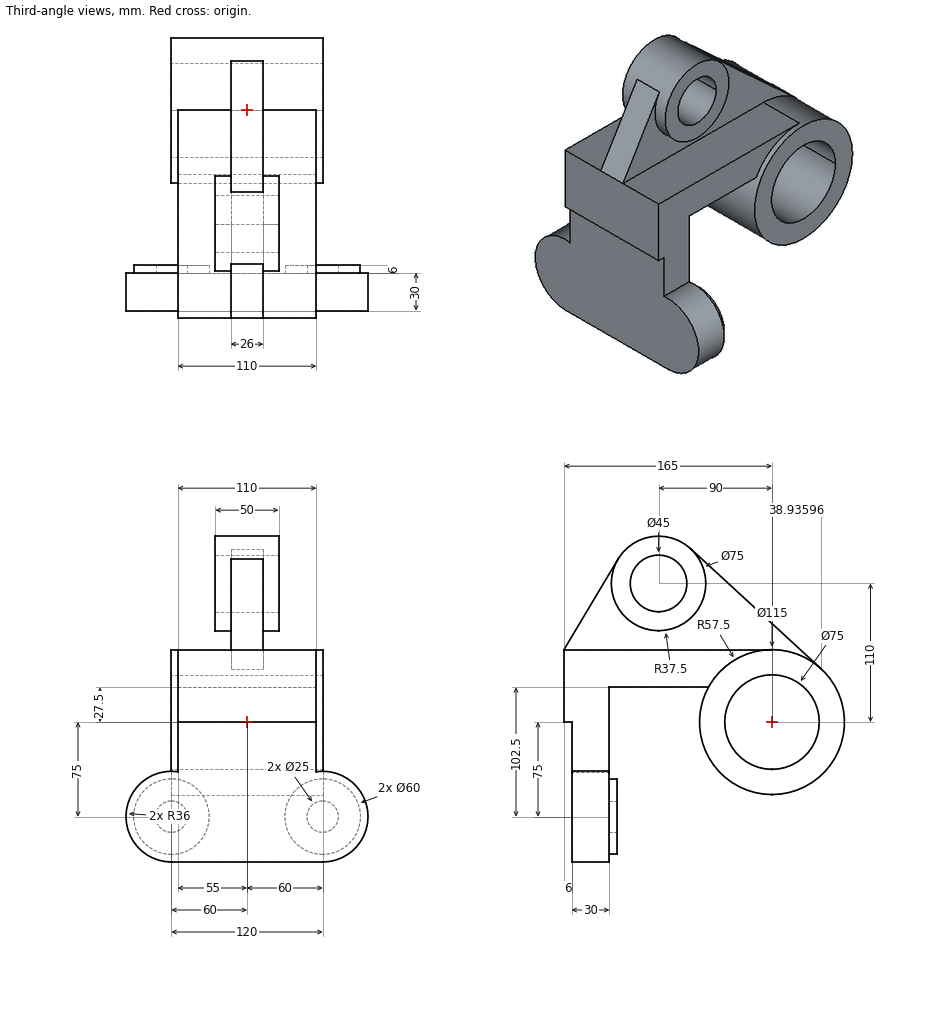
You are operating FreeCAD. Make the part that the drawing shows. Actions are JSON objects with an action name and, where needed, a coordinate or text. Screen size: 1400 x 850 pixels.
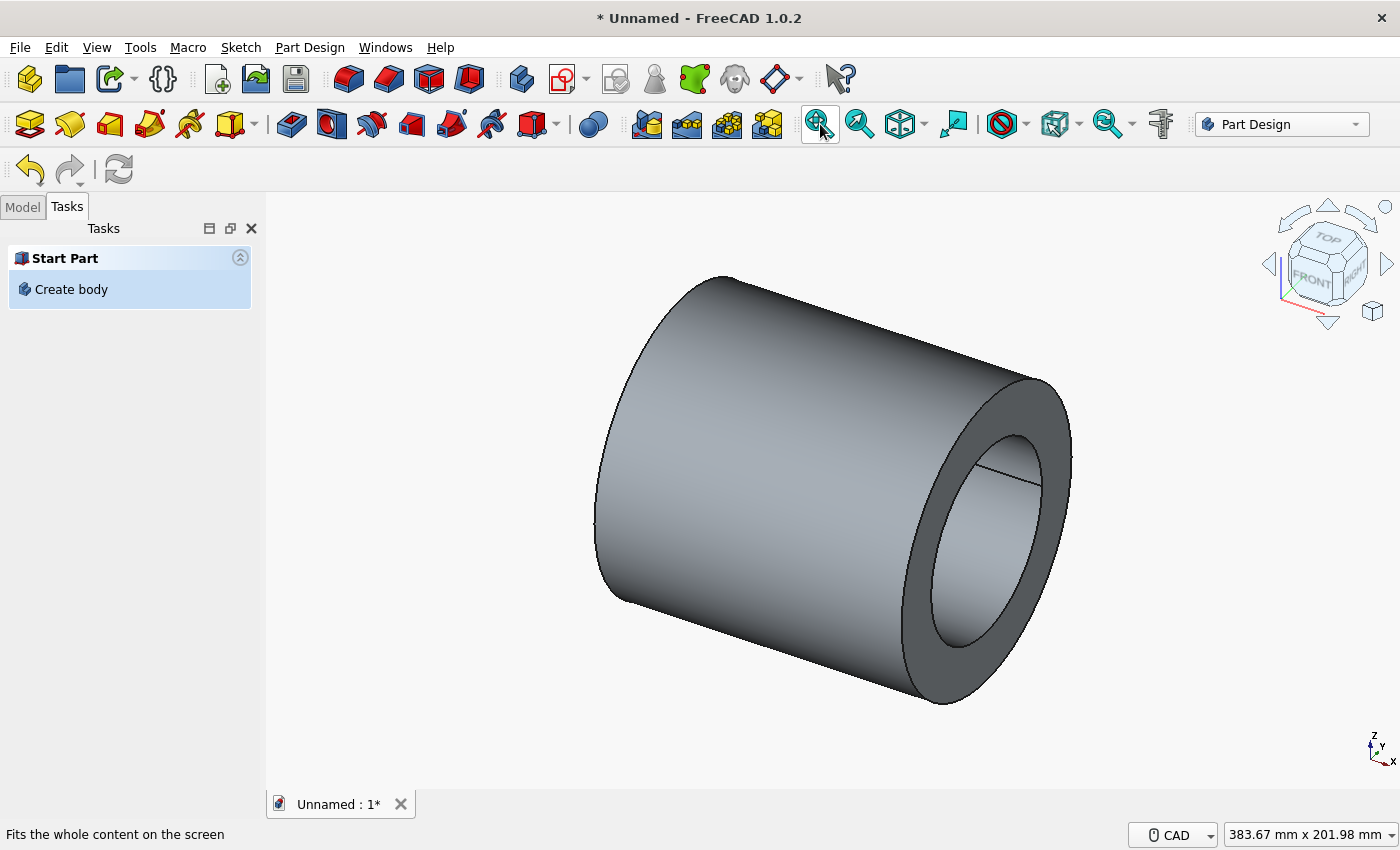
{"action": "left_click", "coordinate": [562, 80]}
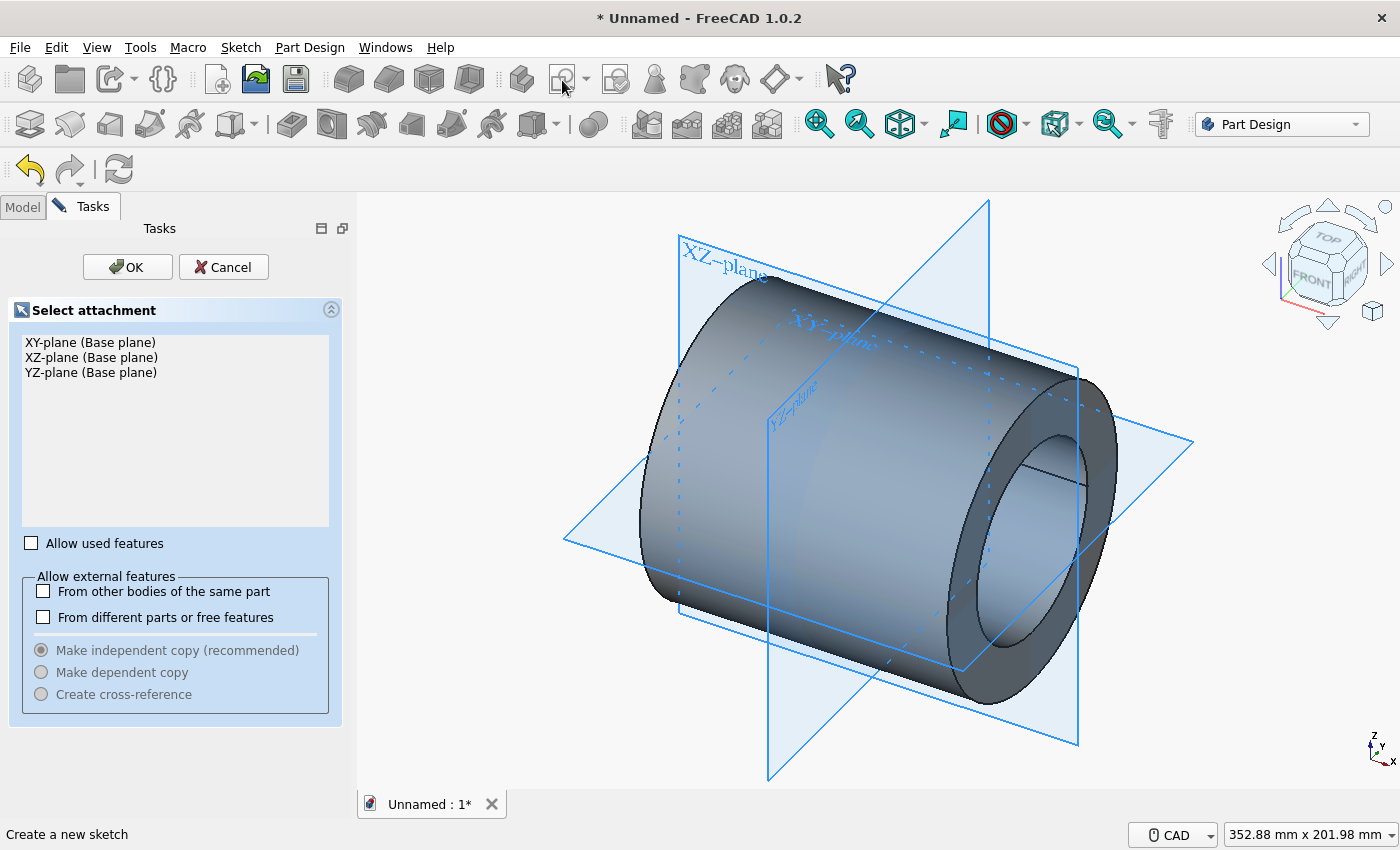
{"action": "left_click", "coordinate": [82, 372]}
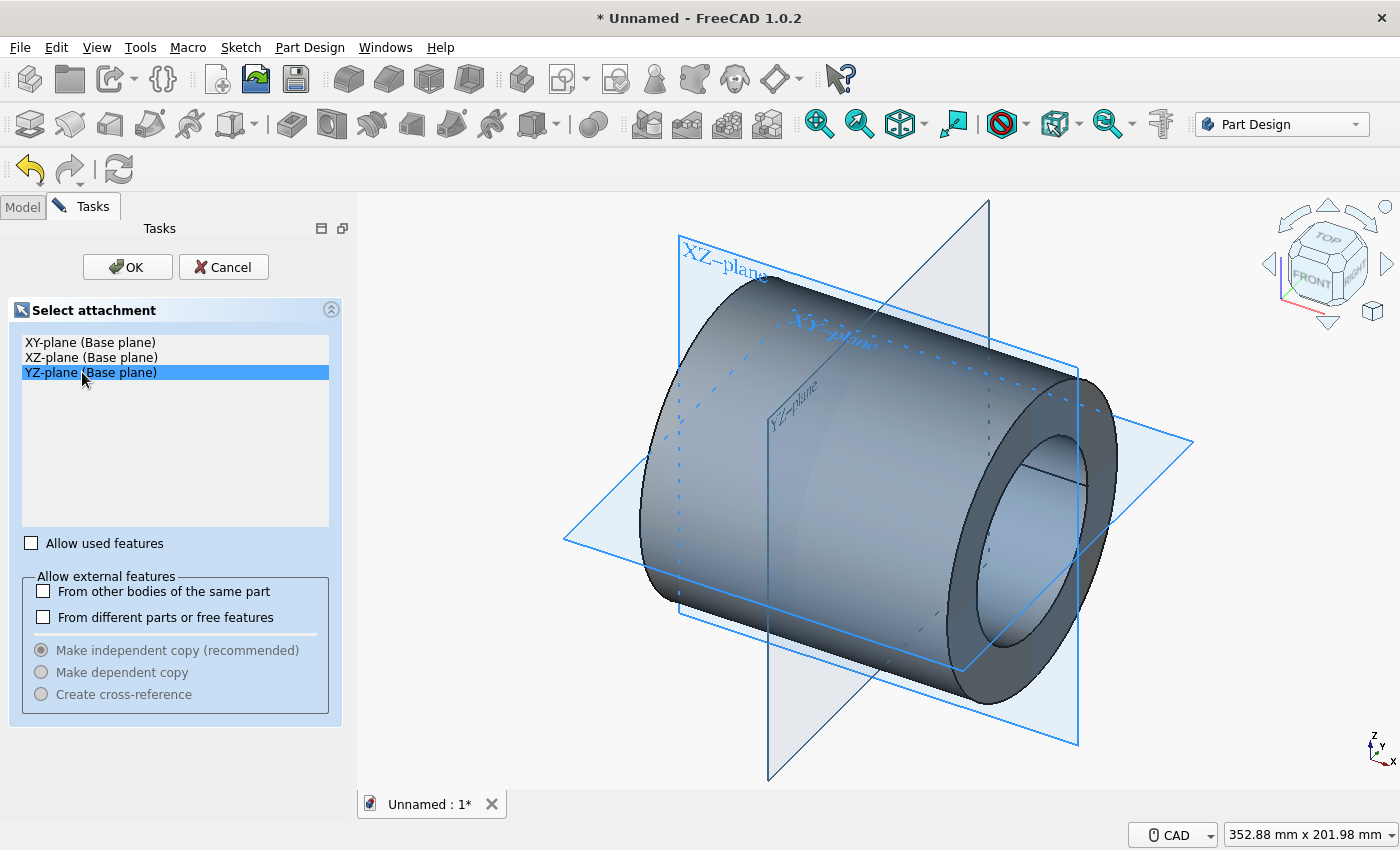
{"action": "left_click", "coordinate": [128, 267]}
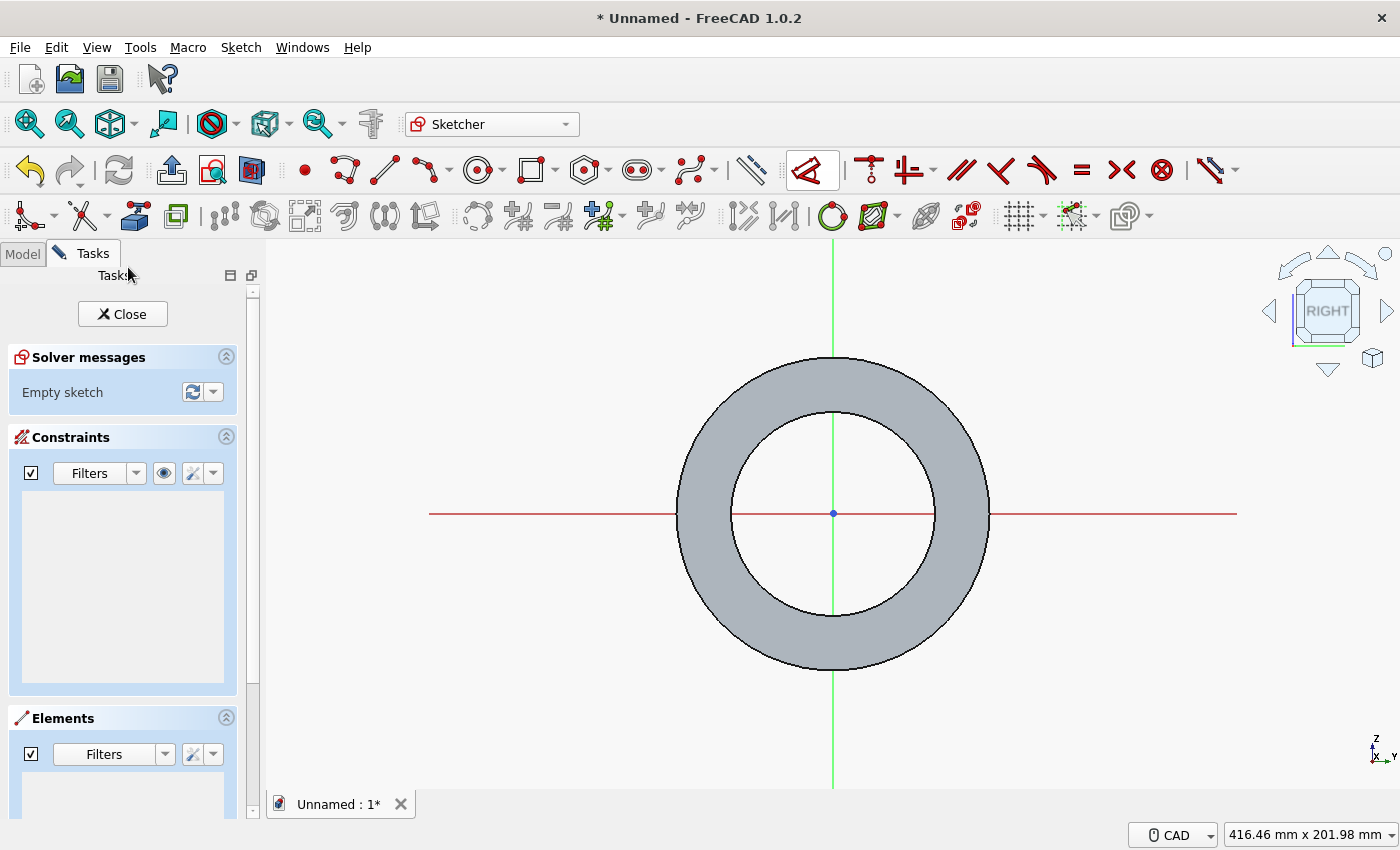
{"action": "left_click", "coordinate": [252, 170]}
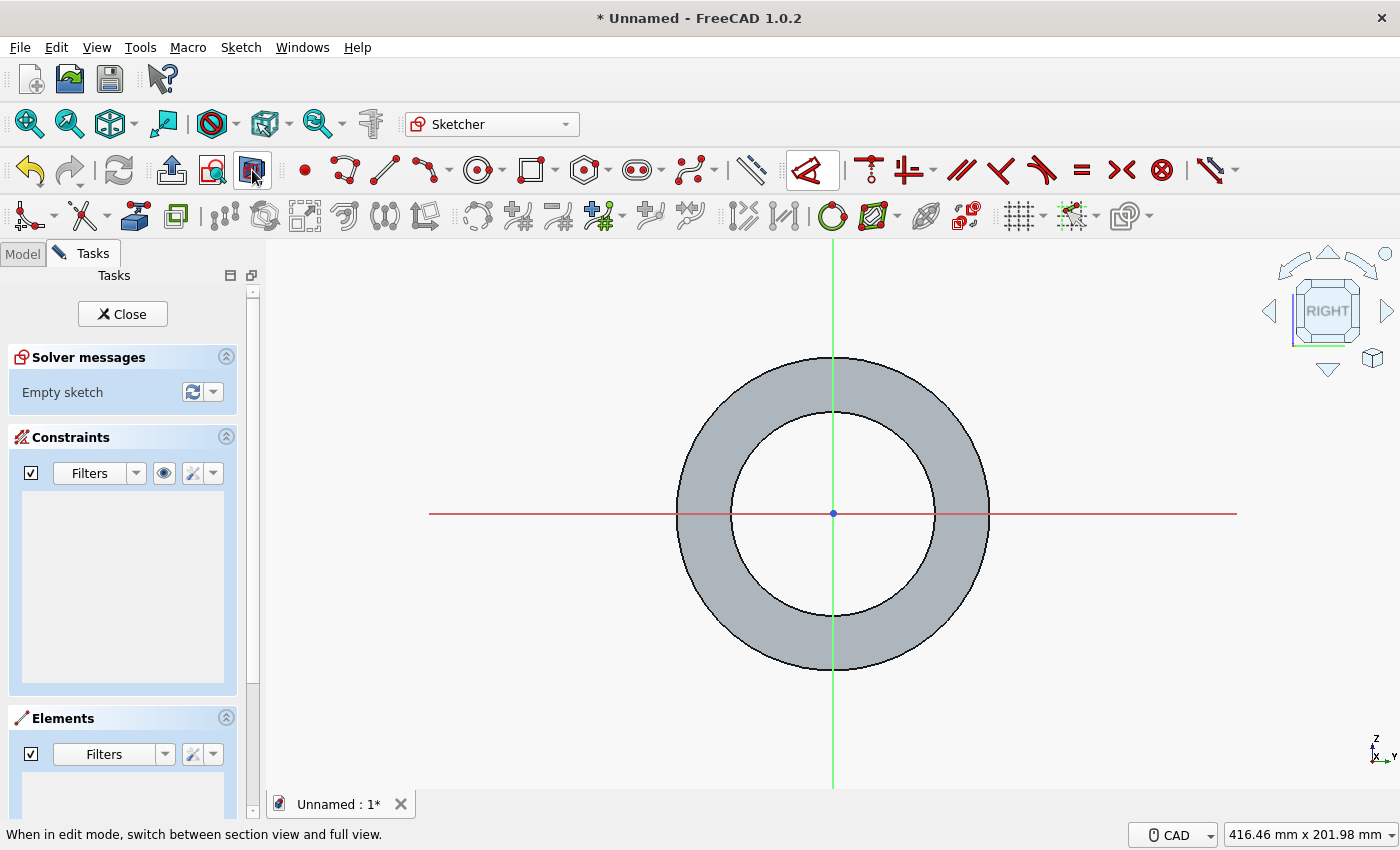
{"action": "key", "text": "g m"}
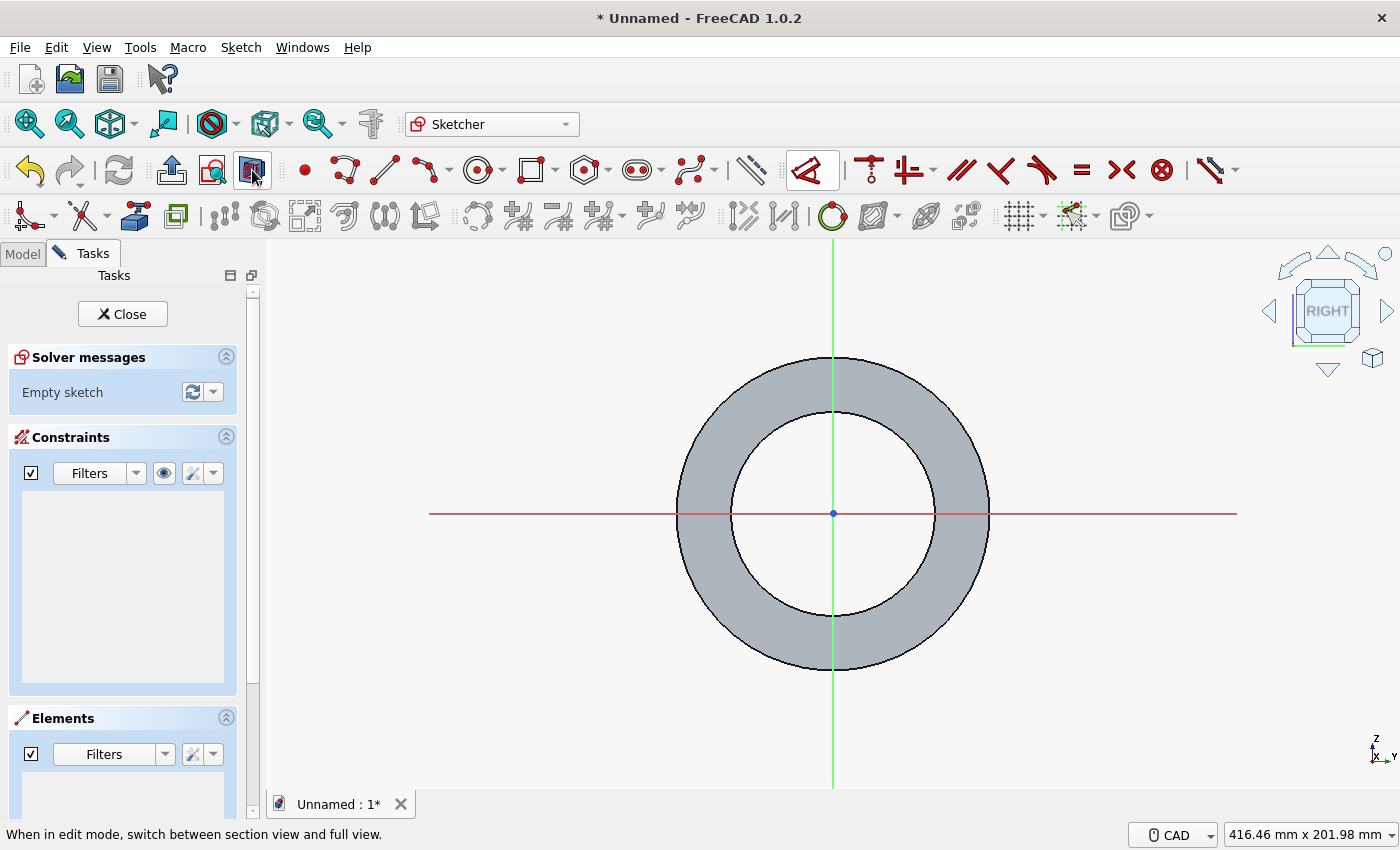
{"action": "left_click", "coordinate": [833, 357]}
{"action": "left_click", "coordinate": [384, 357]}
{"action": "left_click", "coordinate": [384, 514]}
{"action": "left_click", "coordinate": [400, 523]}
{"action": "left_click", "coordinate": [400, 718]}
{"action": "left_click", "coordinate": [482, 718]}
{"action": "left_click", "coordinate": [482, 439]}
{"action": "left_click", "coordinate": [695, 439]}
{"action": "right_click", "coordinate": [695, 439]}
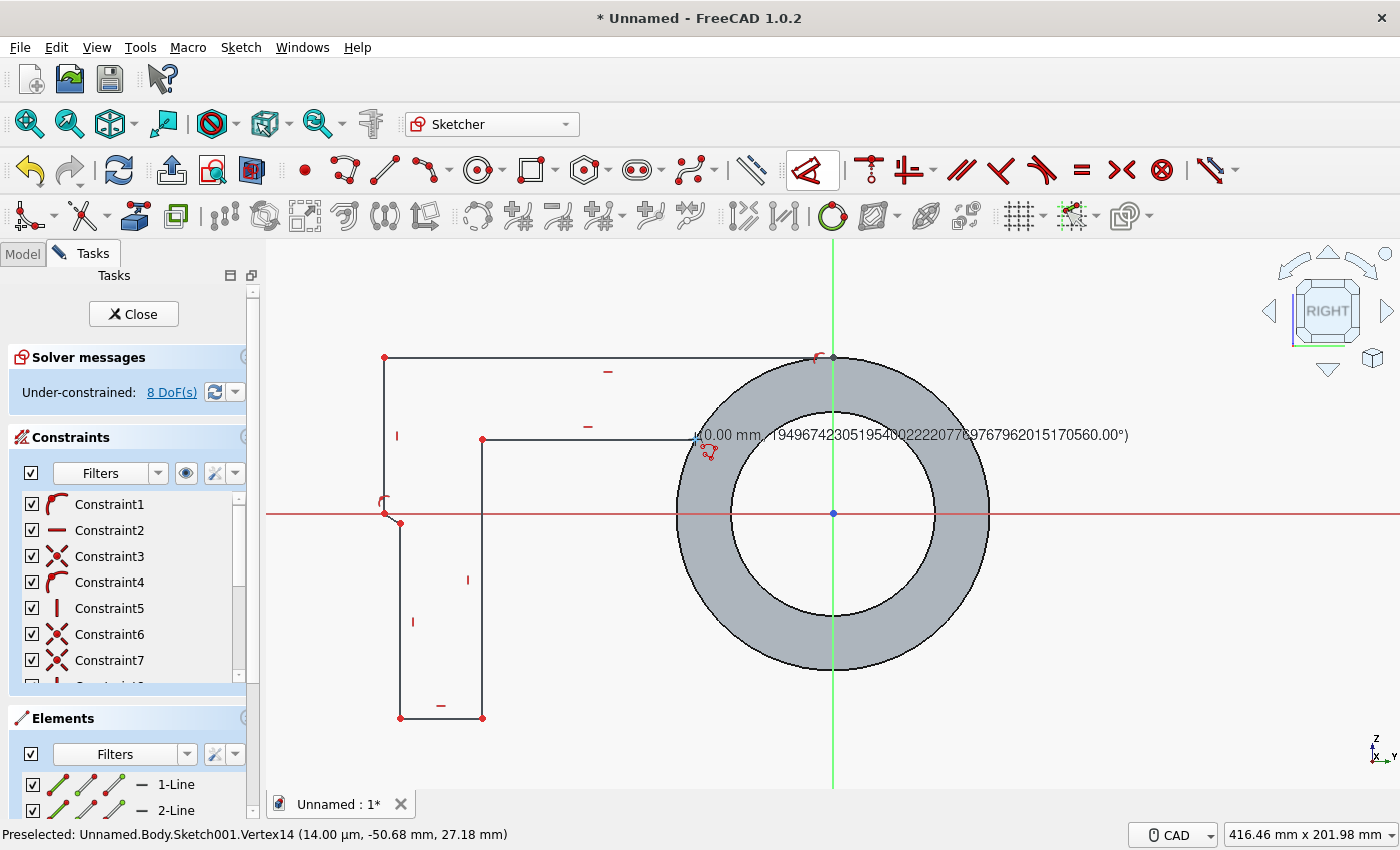
{"action": "left_click", "coordinate": [426, 170]}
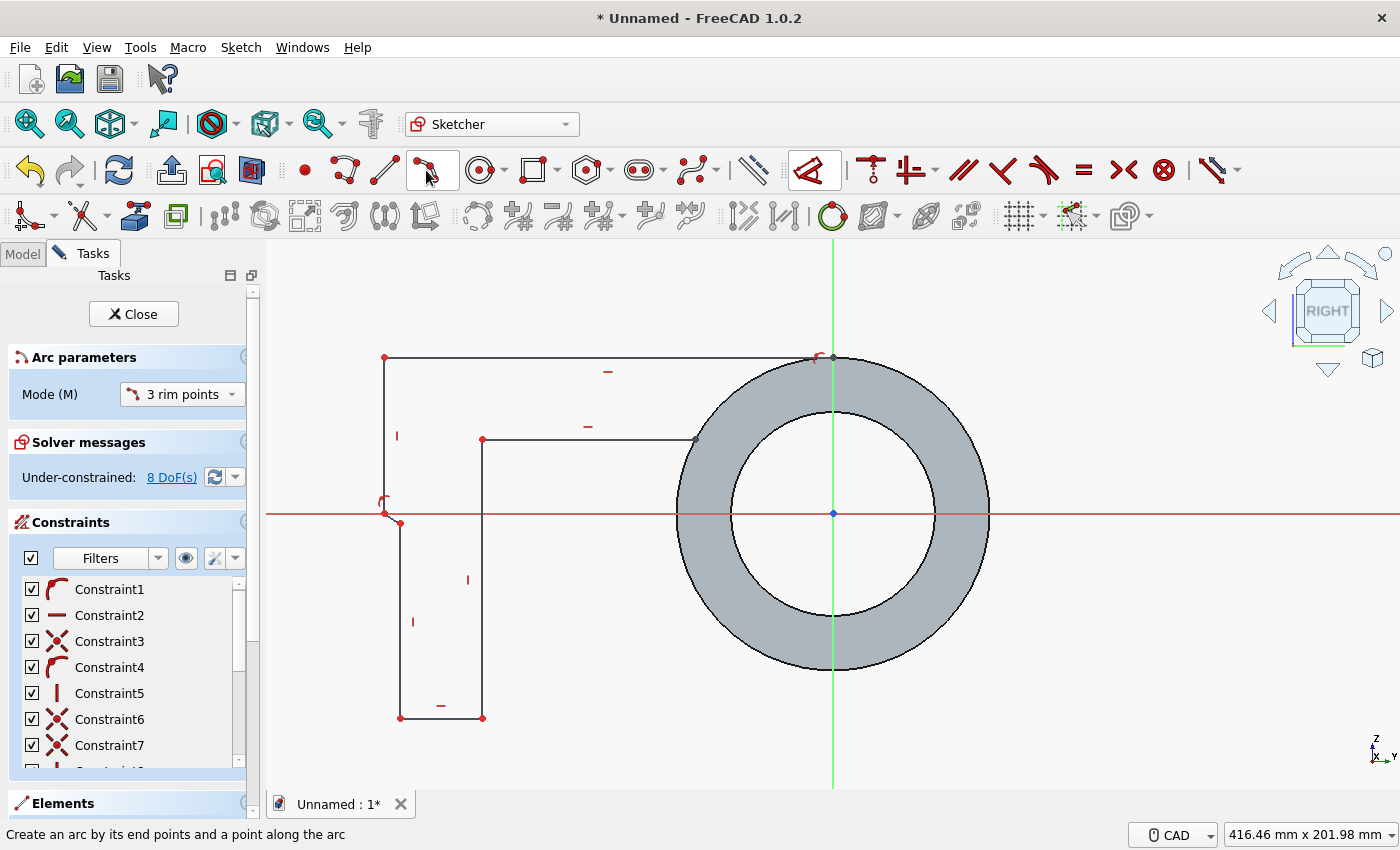
{"action": "left_click", "coordinate": [695, 440]}
{"action": "left_click", "coordinate": [833, 358]}
{"action": "left_click", "coordinate": [753, 379]}
{"action": "key", "text": "Escape"}